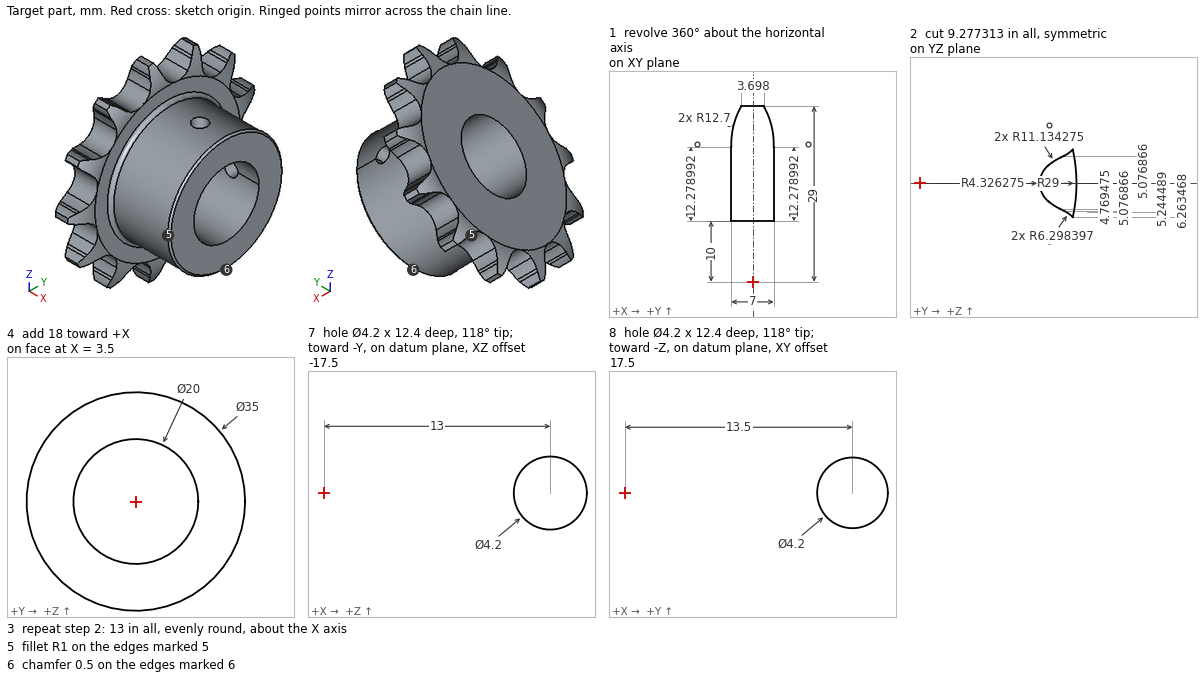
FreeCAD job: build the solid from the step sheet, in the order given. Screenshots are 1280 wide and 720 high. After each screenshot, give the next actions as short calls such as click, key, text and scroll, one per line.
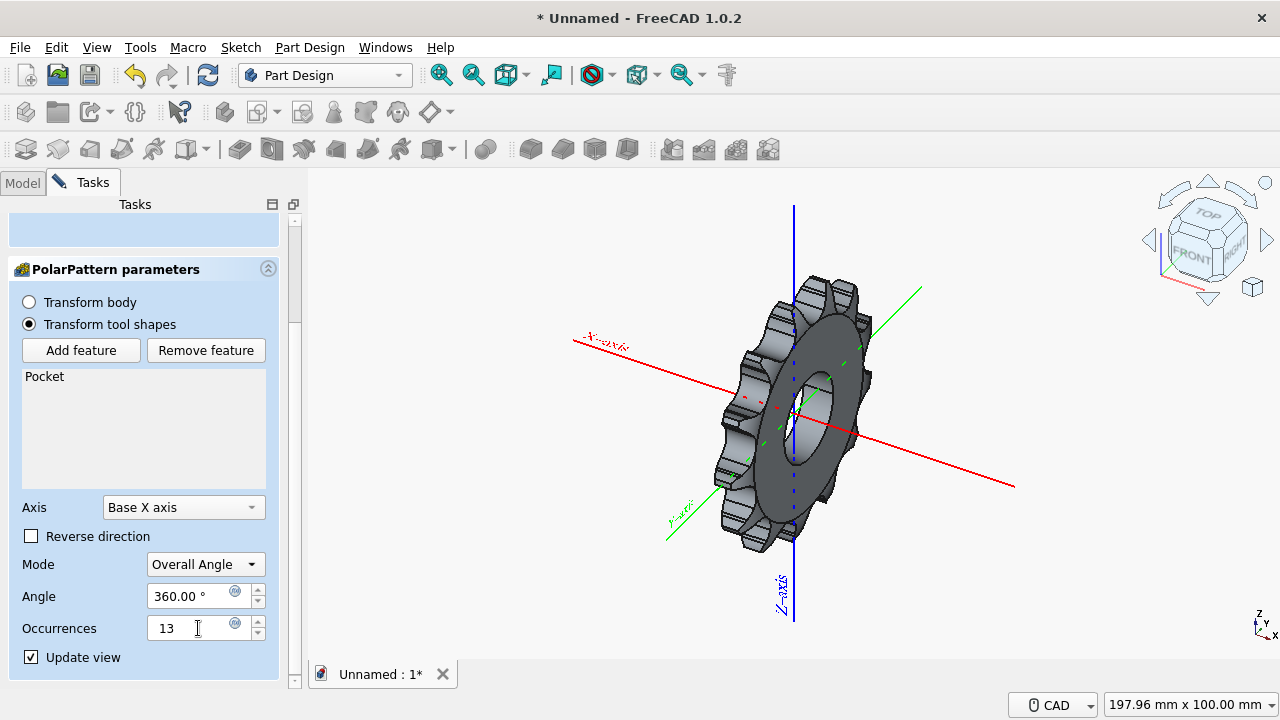
scroll(295, 451, up, 3)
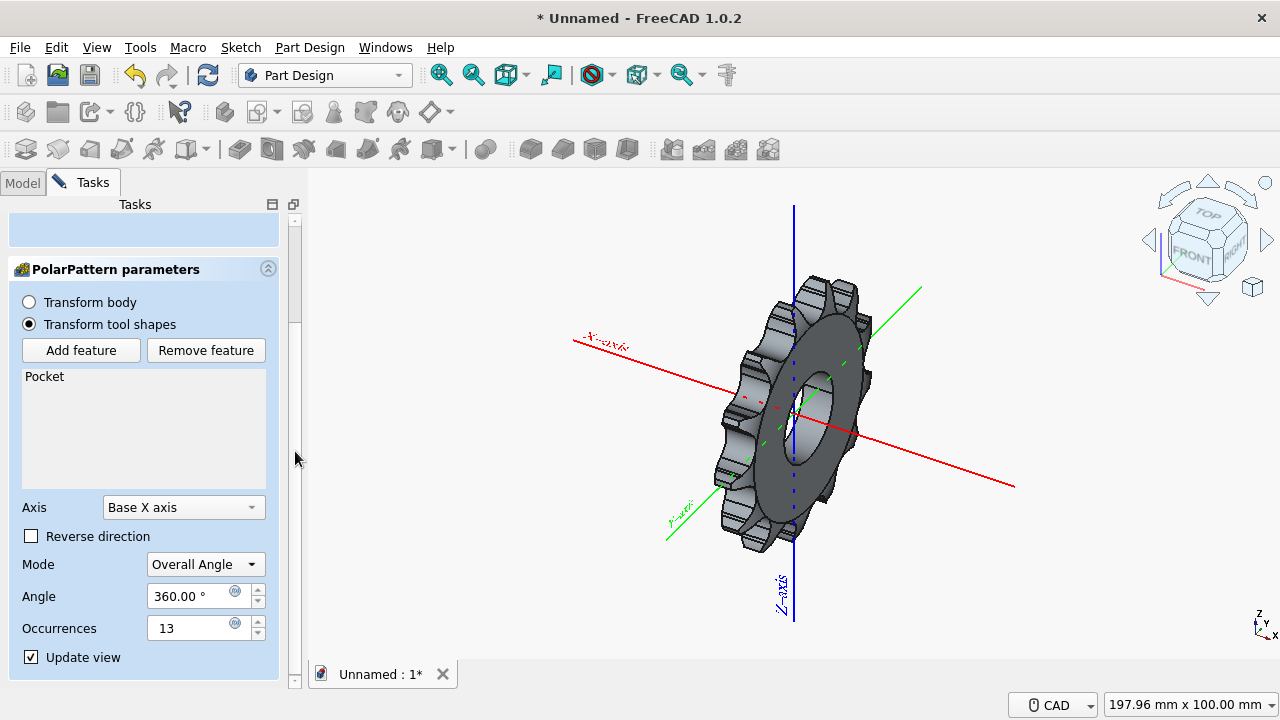
click(96, 243)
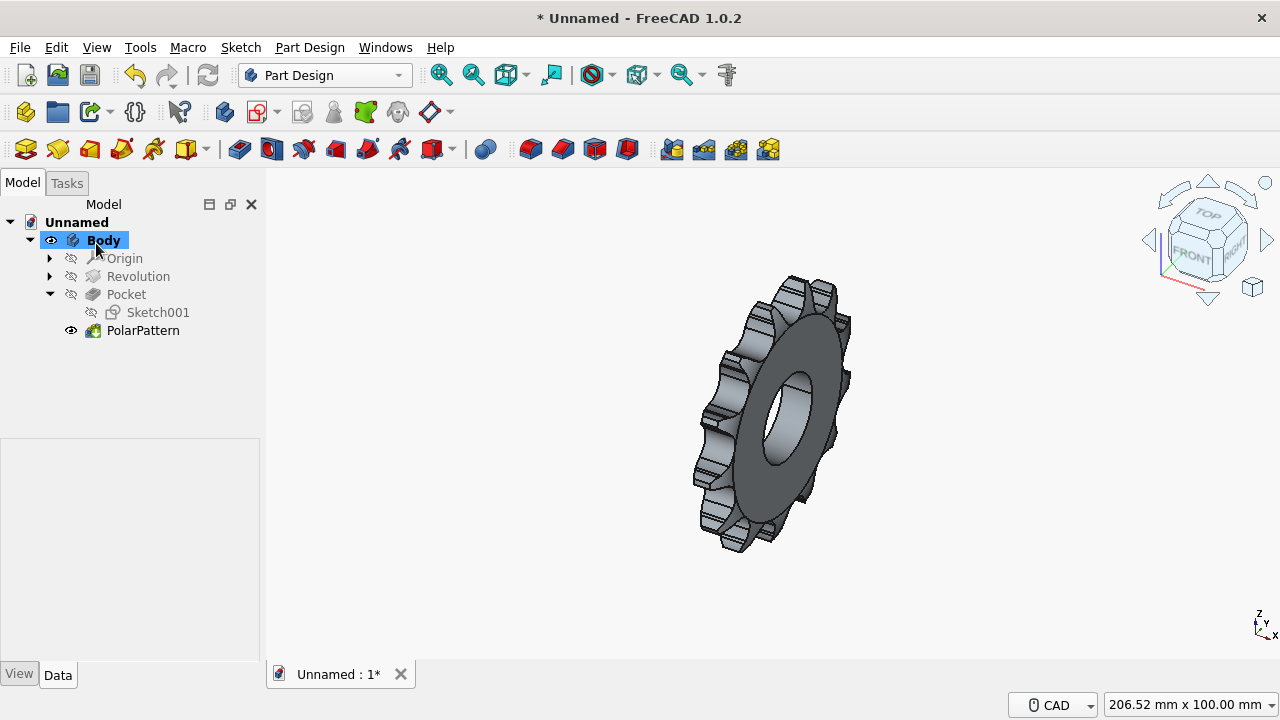
click(819, 335)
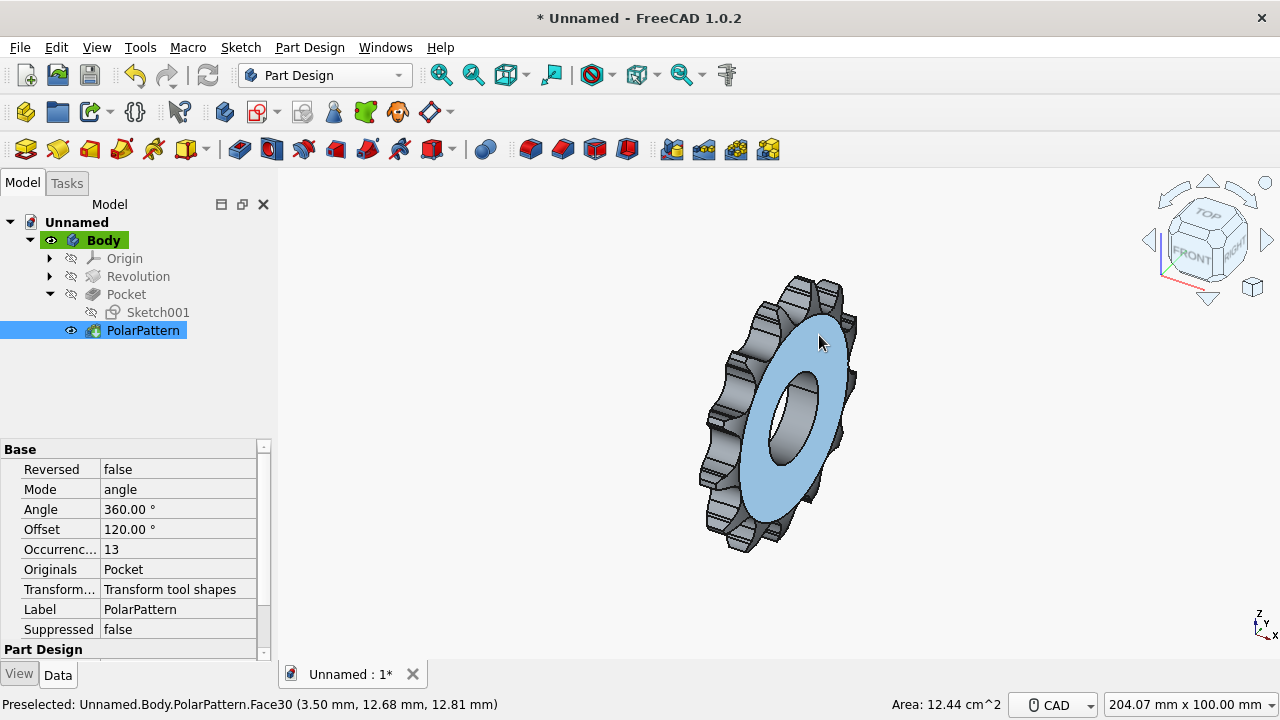
click(258, 112)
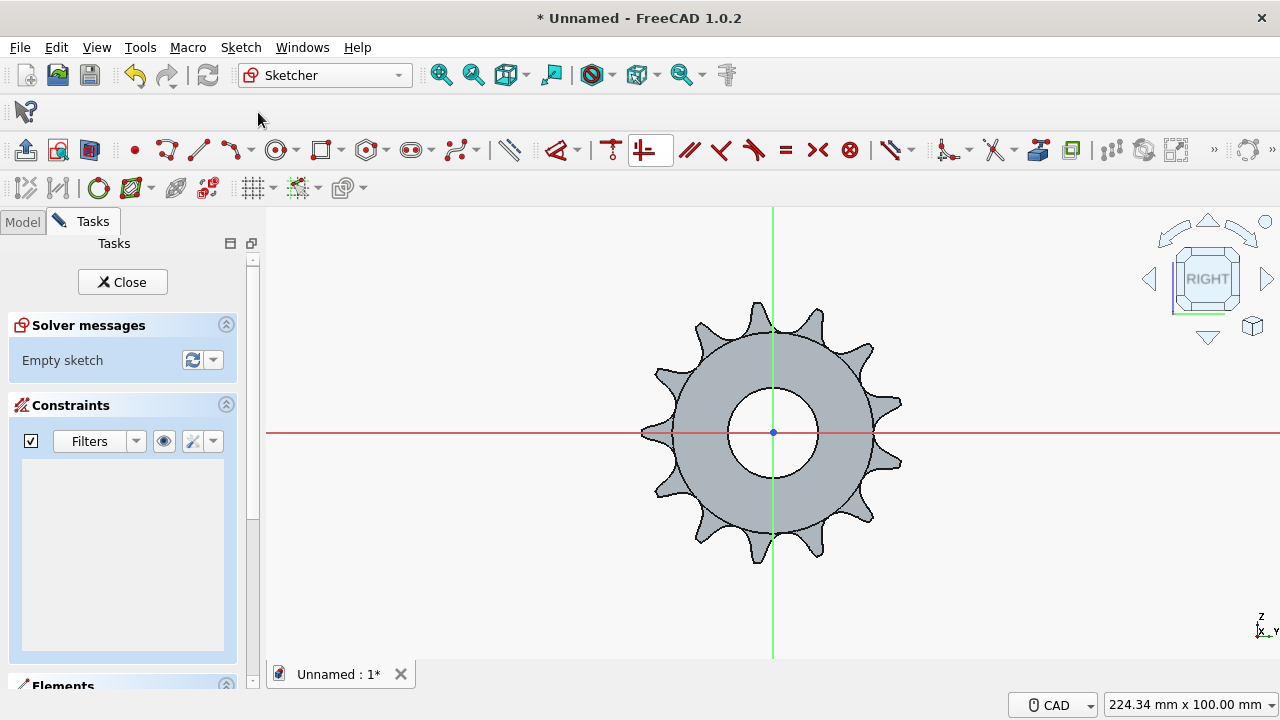
scroll(856, 433, up, 3)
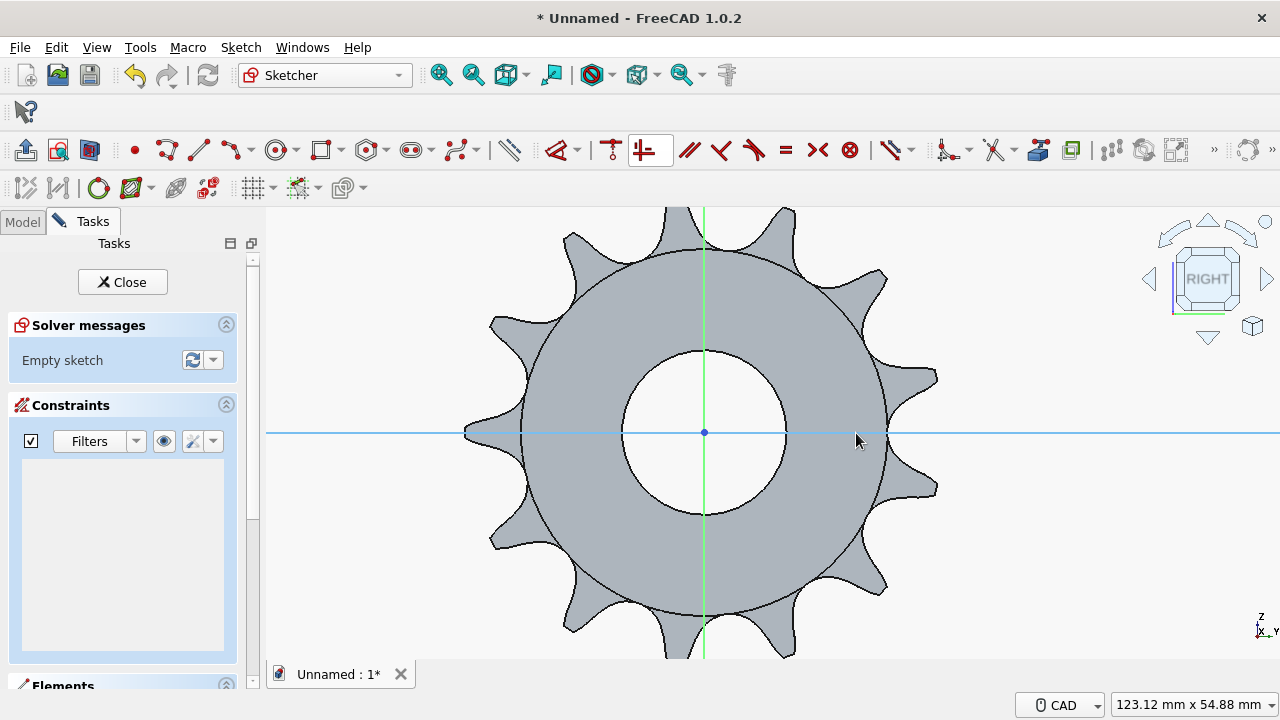
click(276, 150)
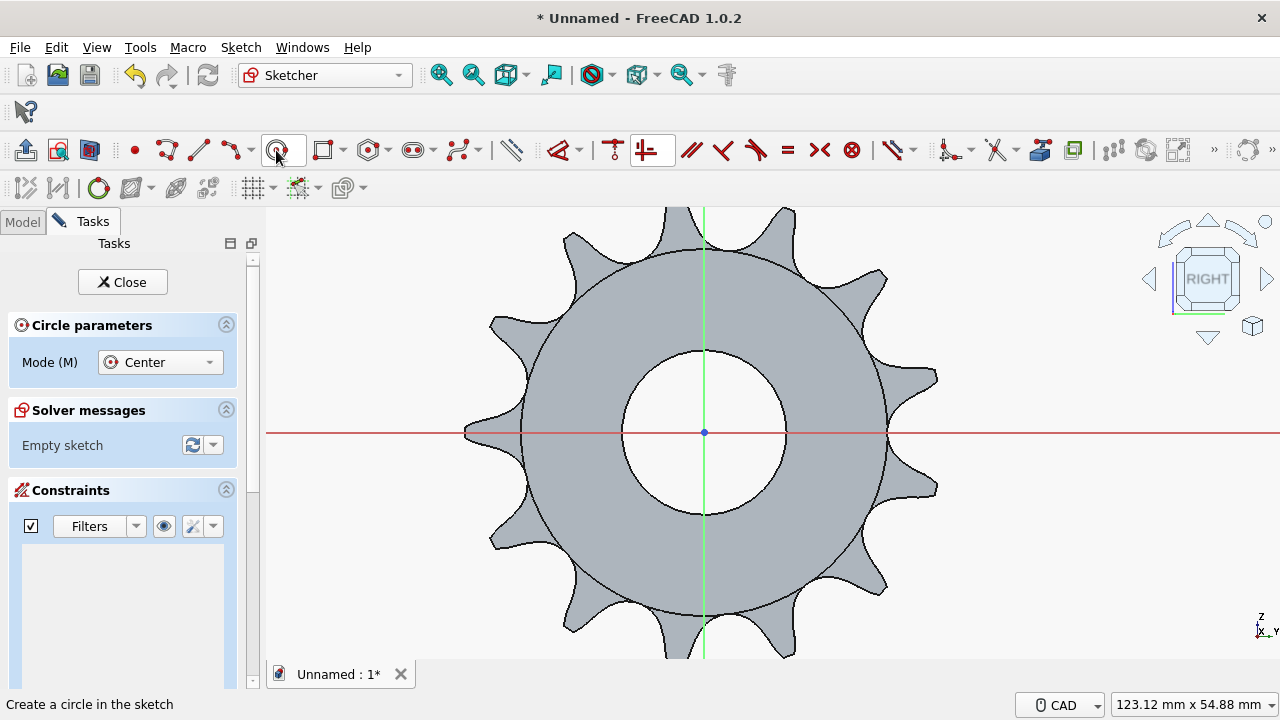
click(704, 433)
move(806, 331)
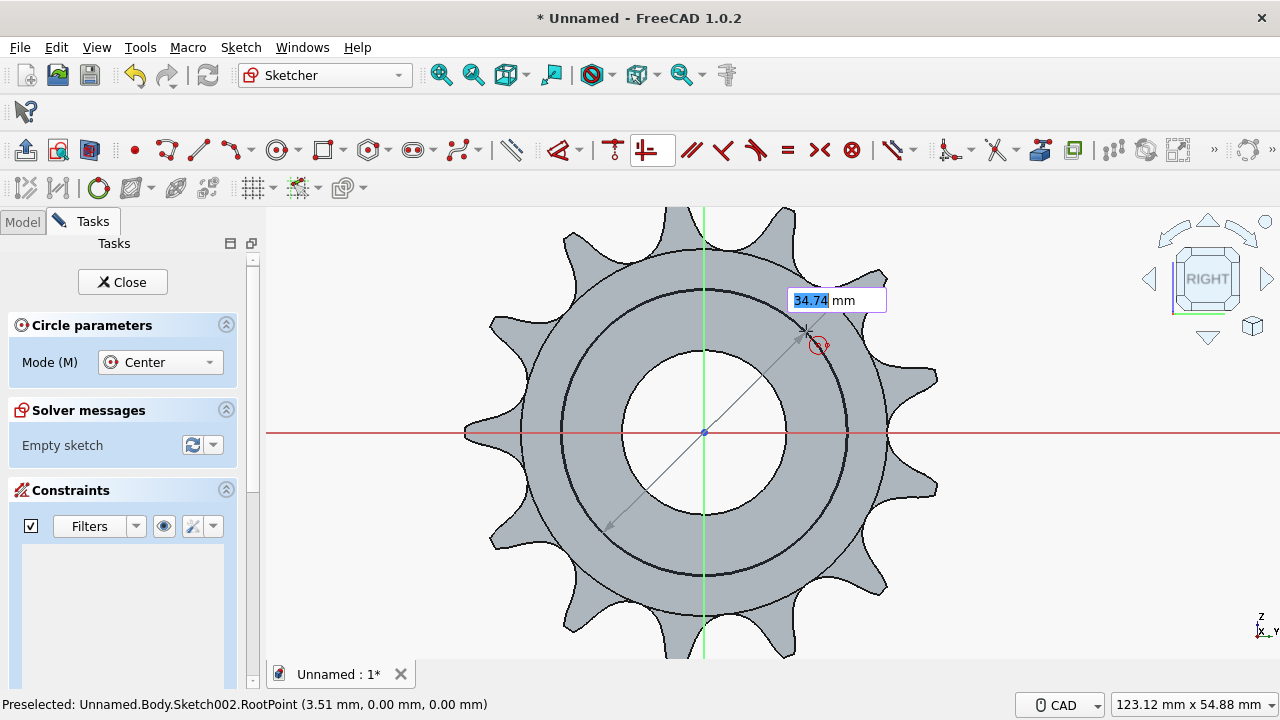
text(35)
key(Return)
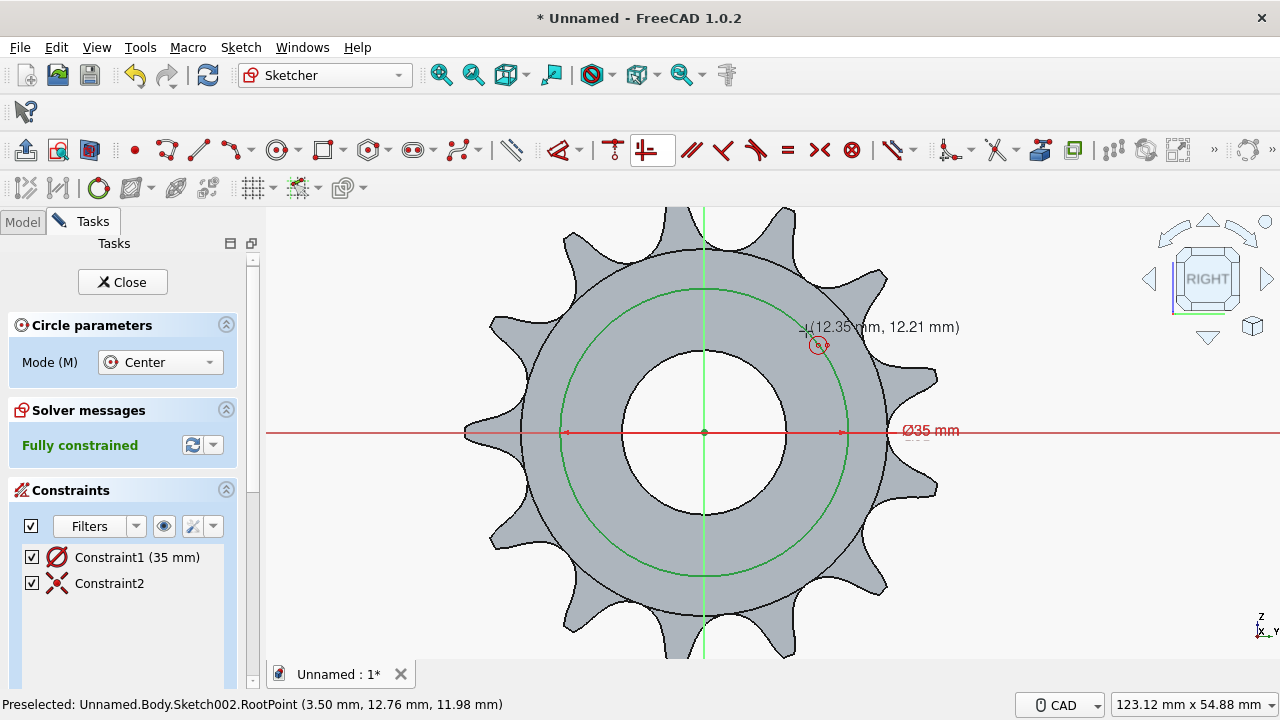
click(704, 433)
move(763, 374)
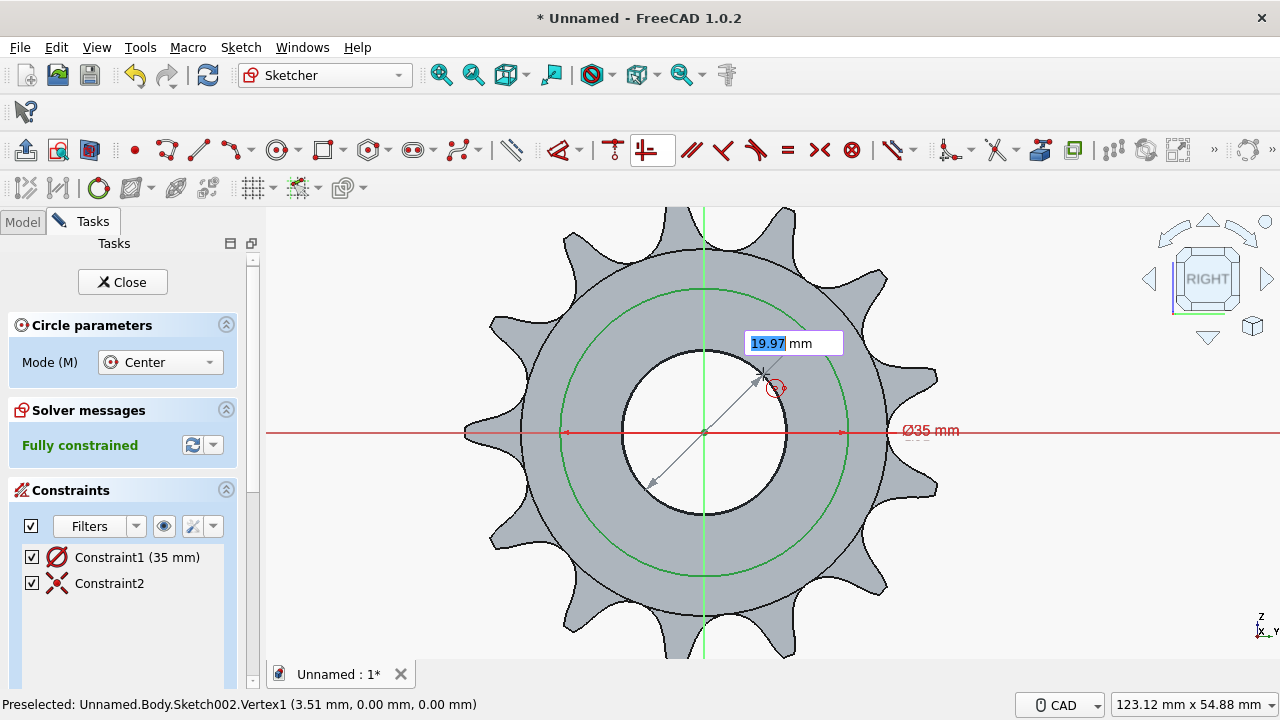
text(20)
key(Return)
key(Escape)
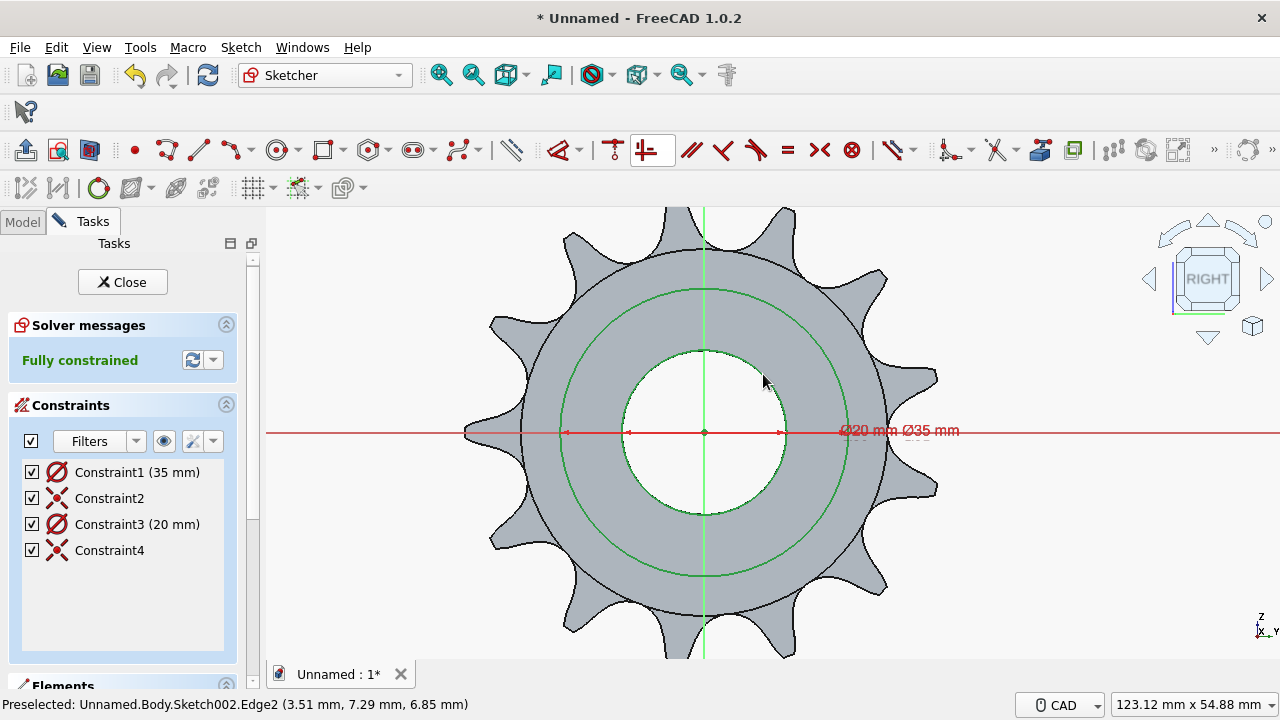
click(123, 282)